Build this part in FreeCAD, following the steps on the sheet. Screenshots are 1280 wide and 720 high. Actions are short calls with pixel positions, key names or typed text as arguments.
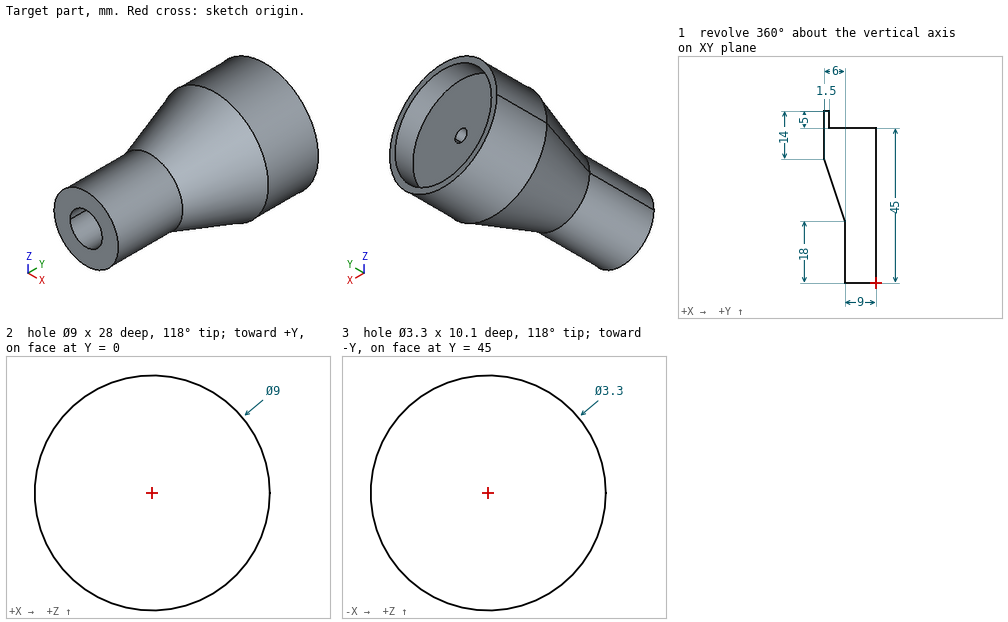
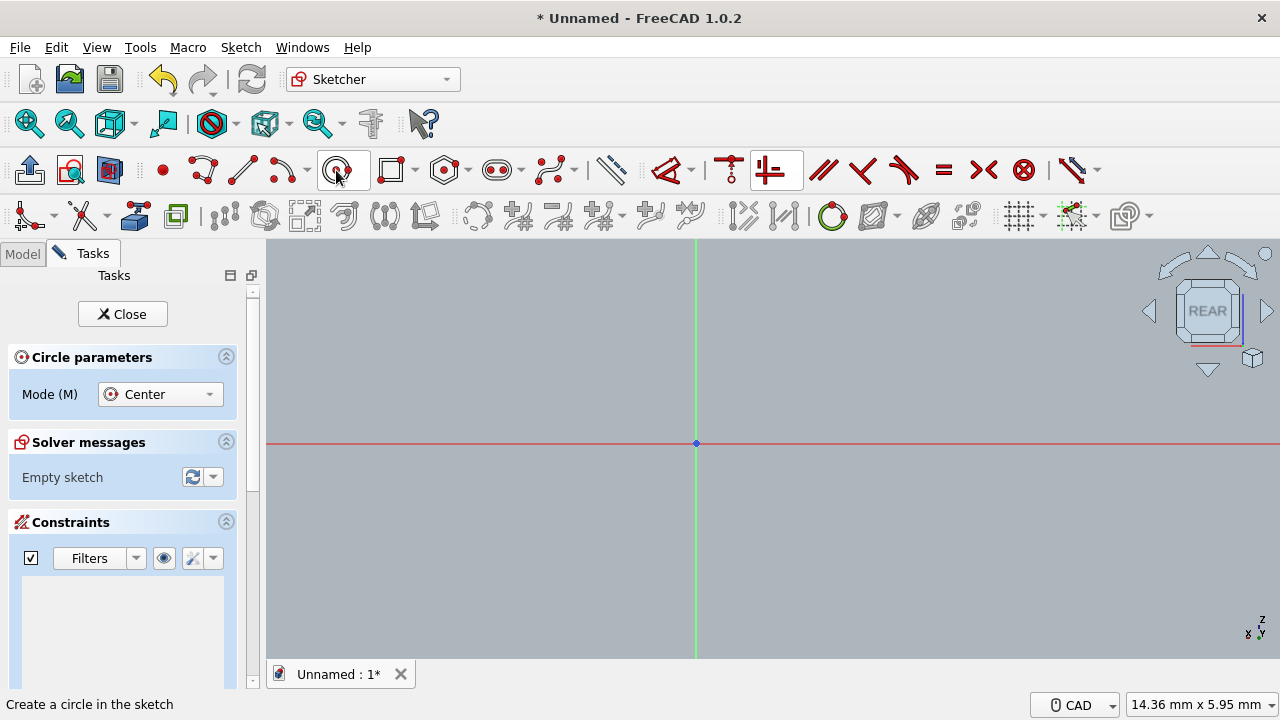
click(696, 444)
move(779, 362)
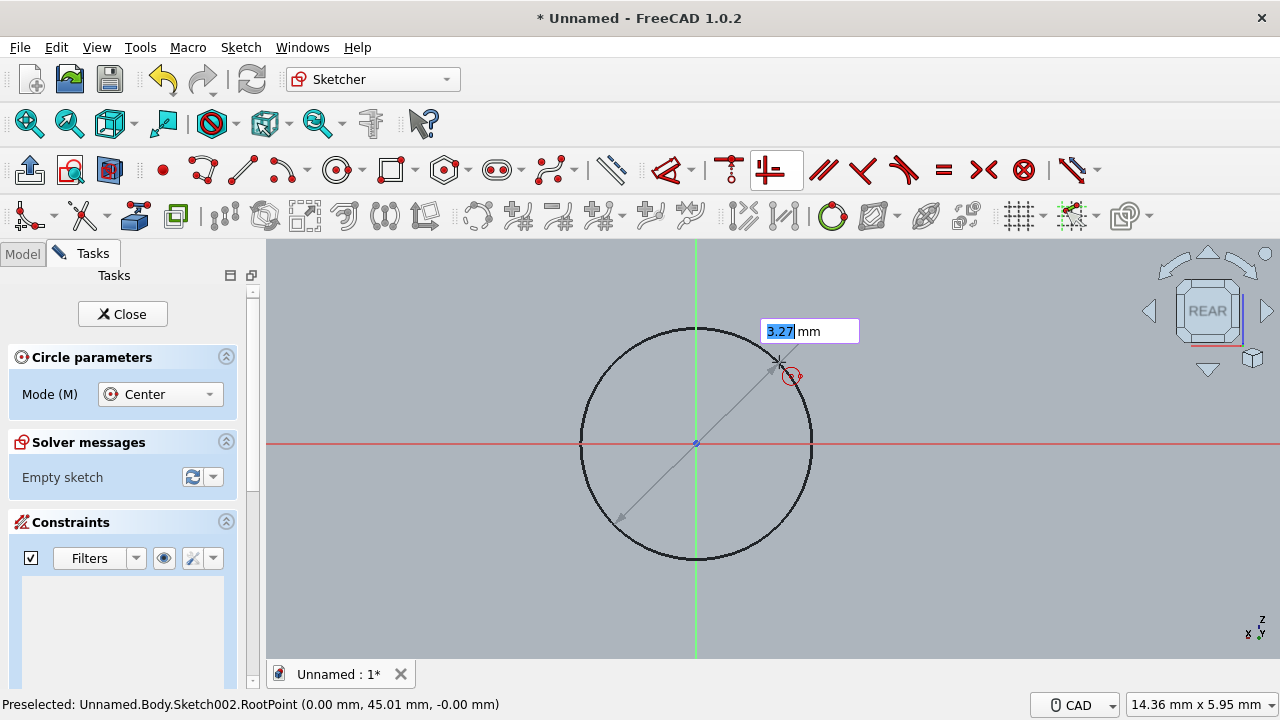
text(3.3)
key(Return)
key(Escape)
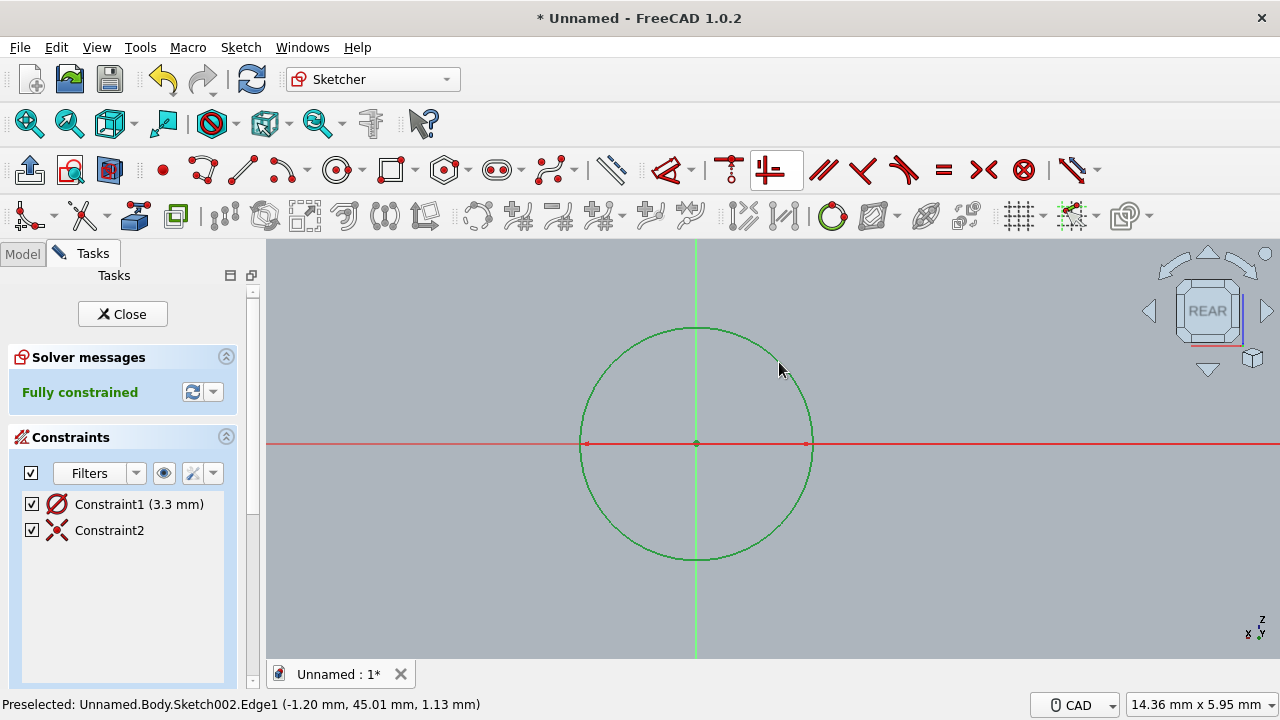
click(123, 314)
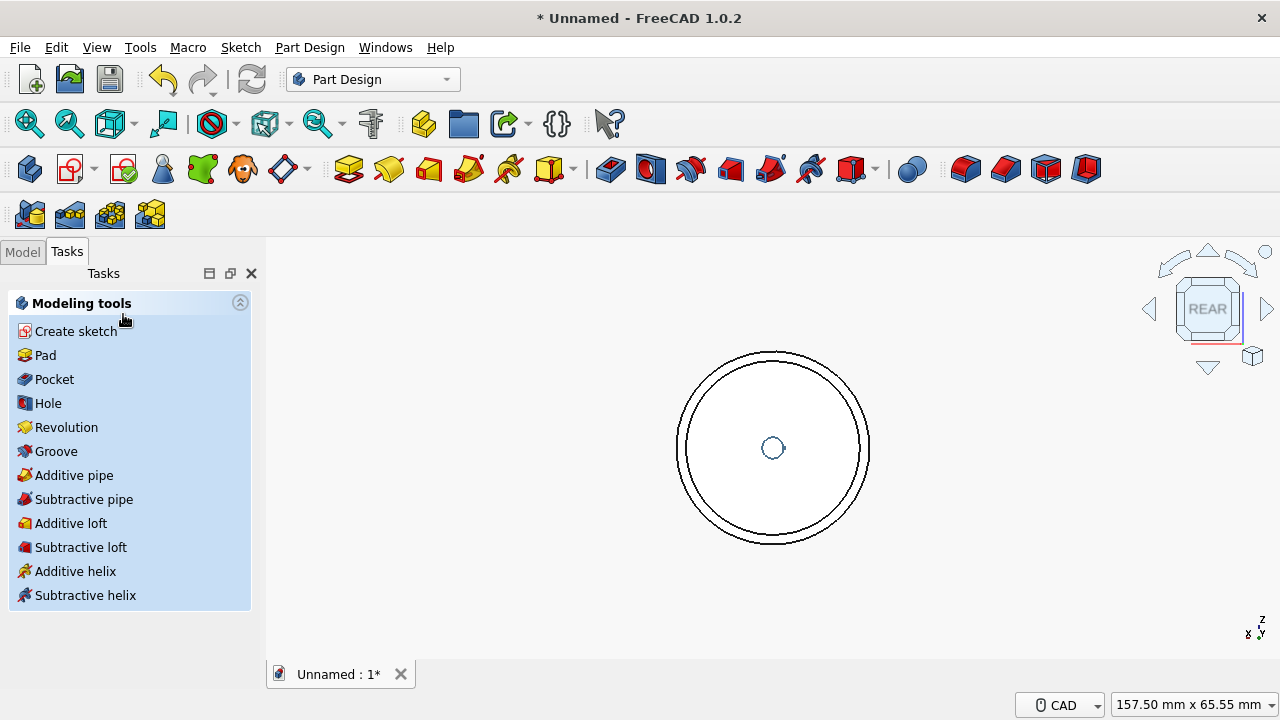
click(652, 170)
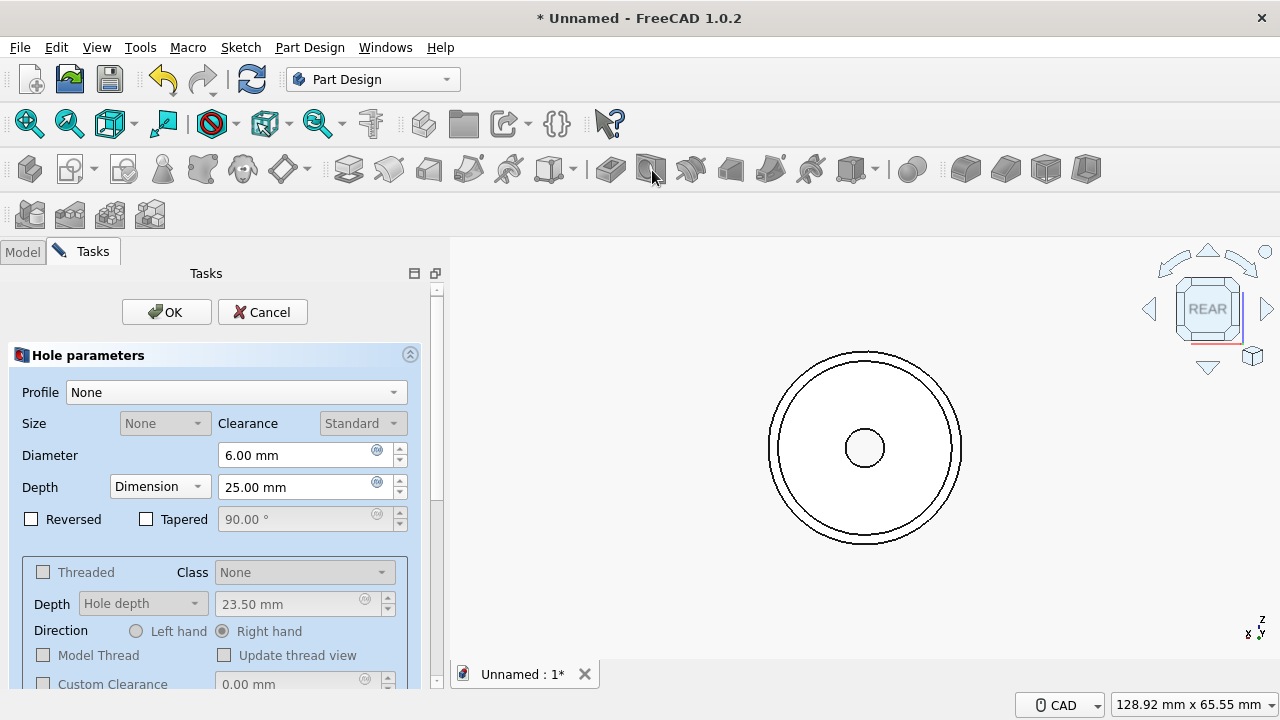
triple_click(305, 455)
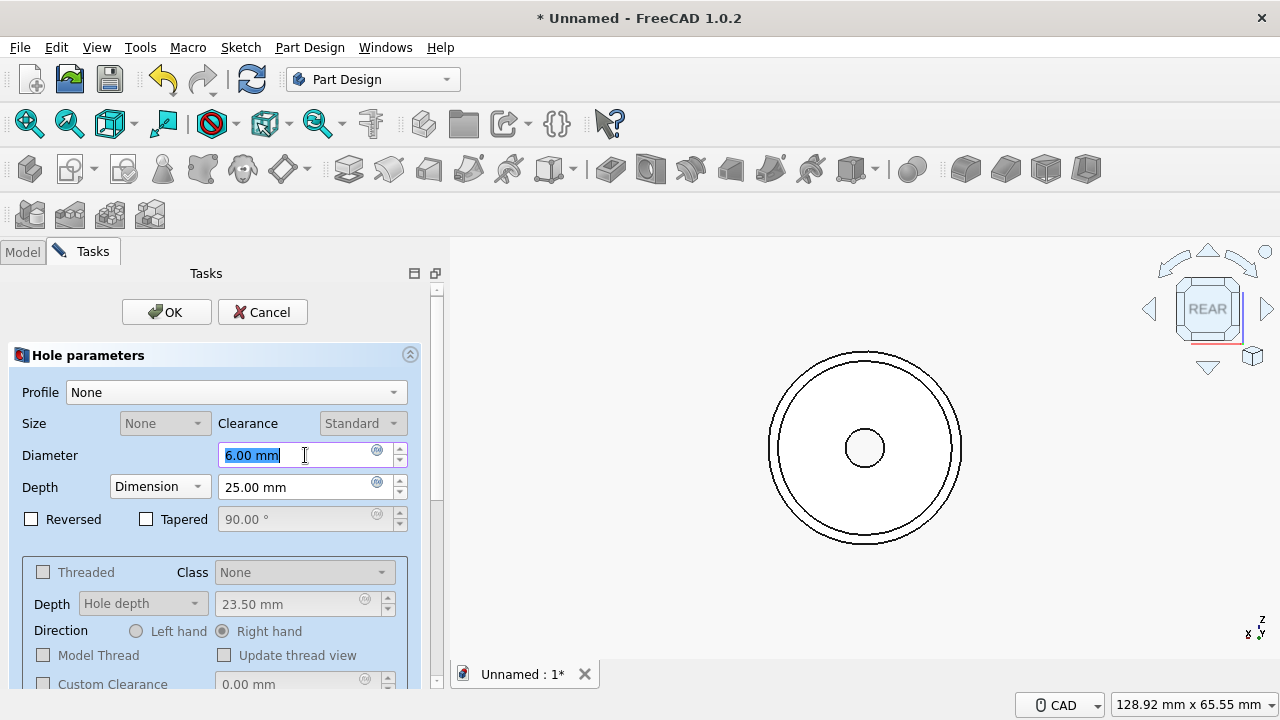
text(3.3)
key(Tab)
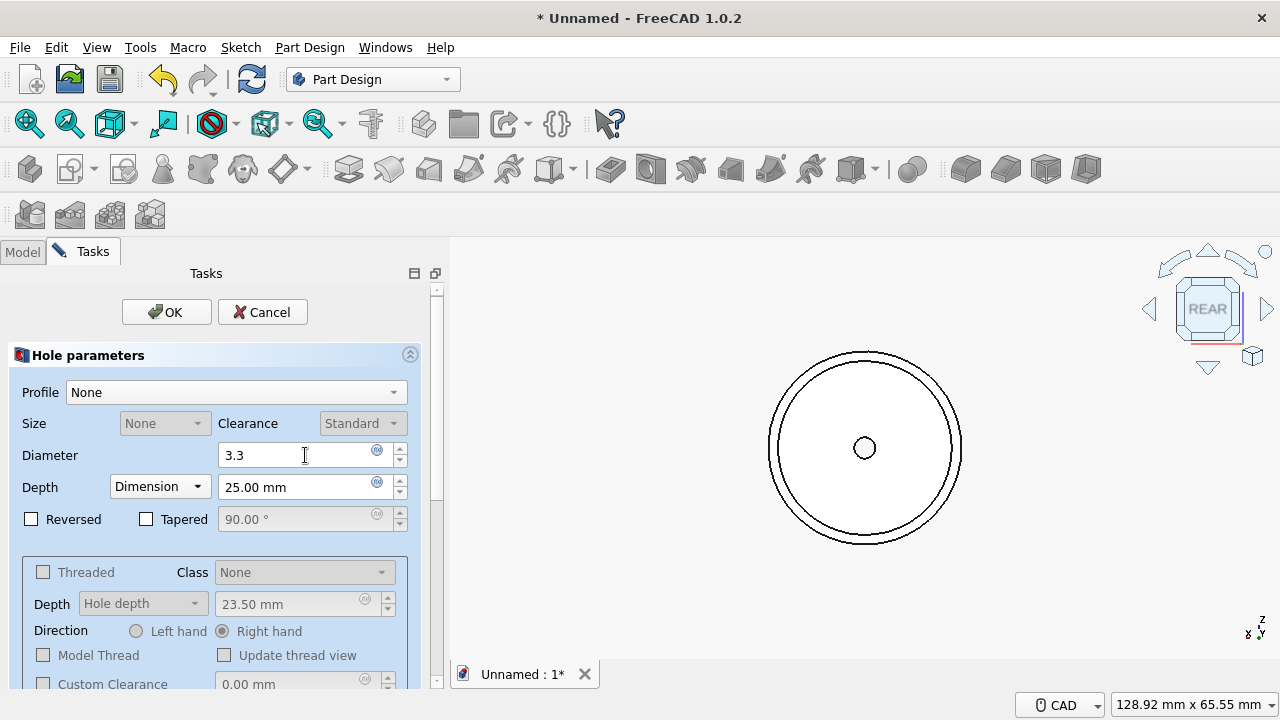
triple_click(305, 487)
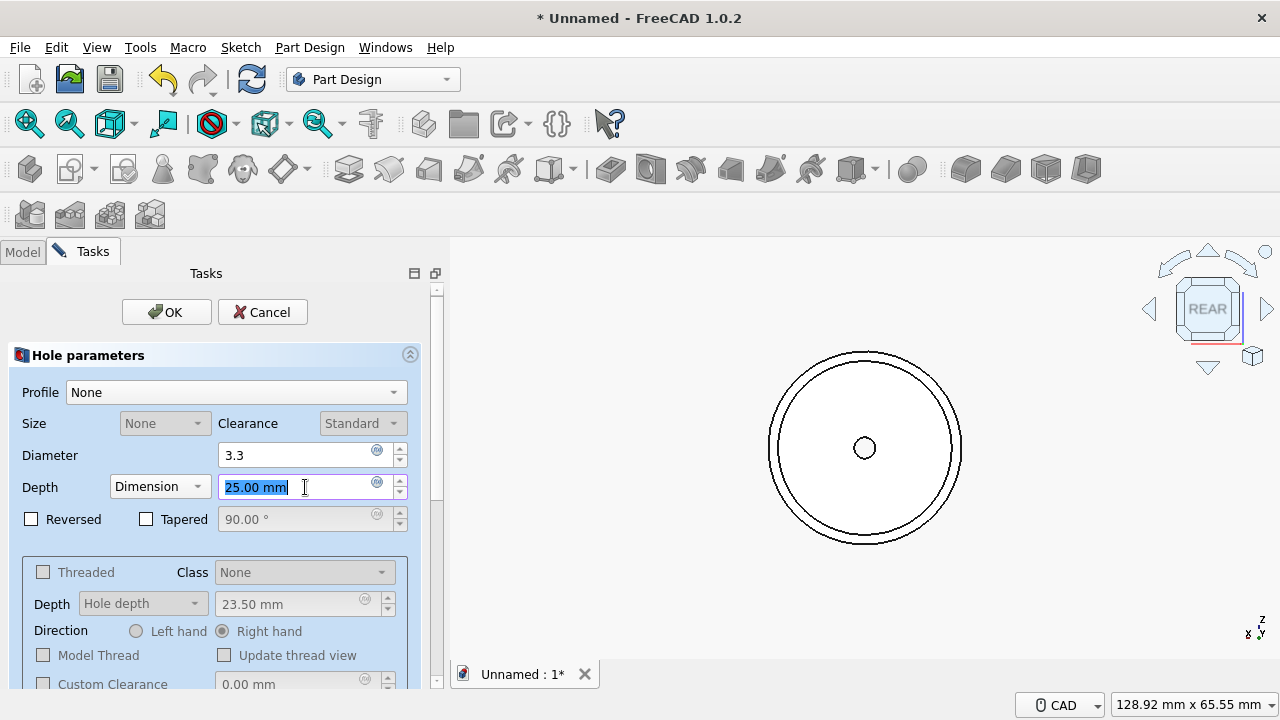
text(10.1)
key(Tab)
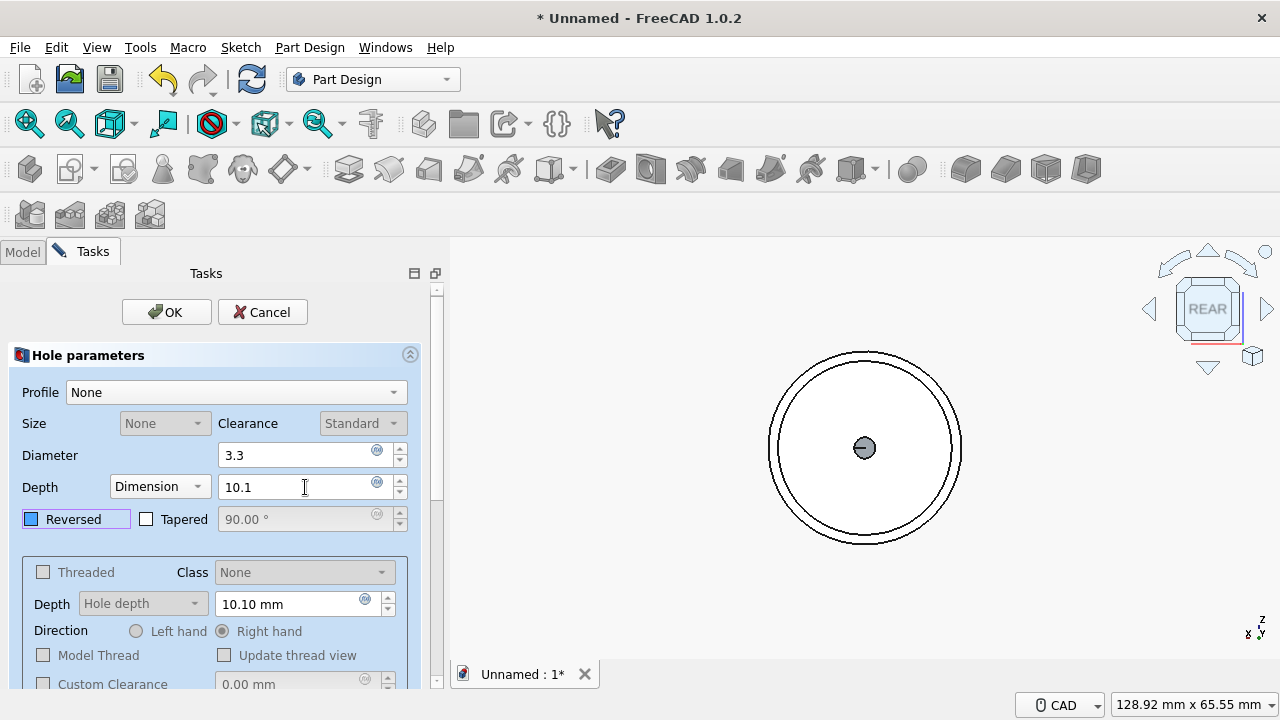
click(167, 312)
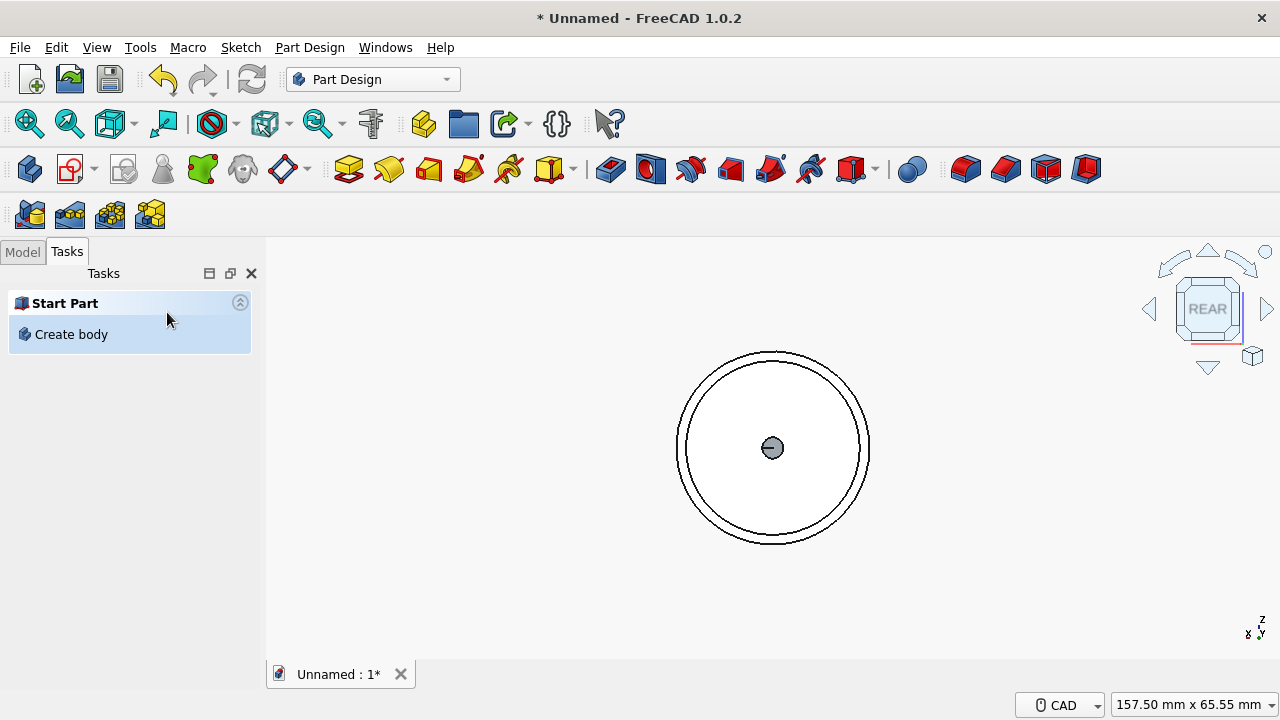
key(0)